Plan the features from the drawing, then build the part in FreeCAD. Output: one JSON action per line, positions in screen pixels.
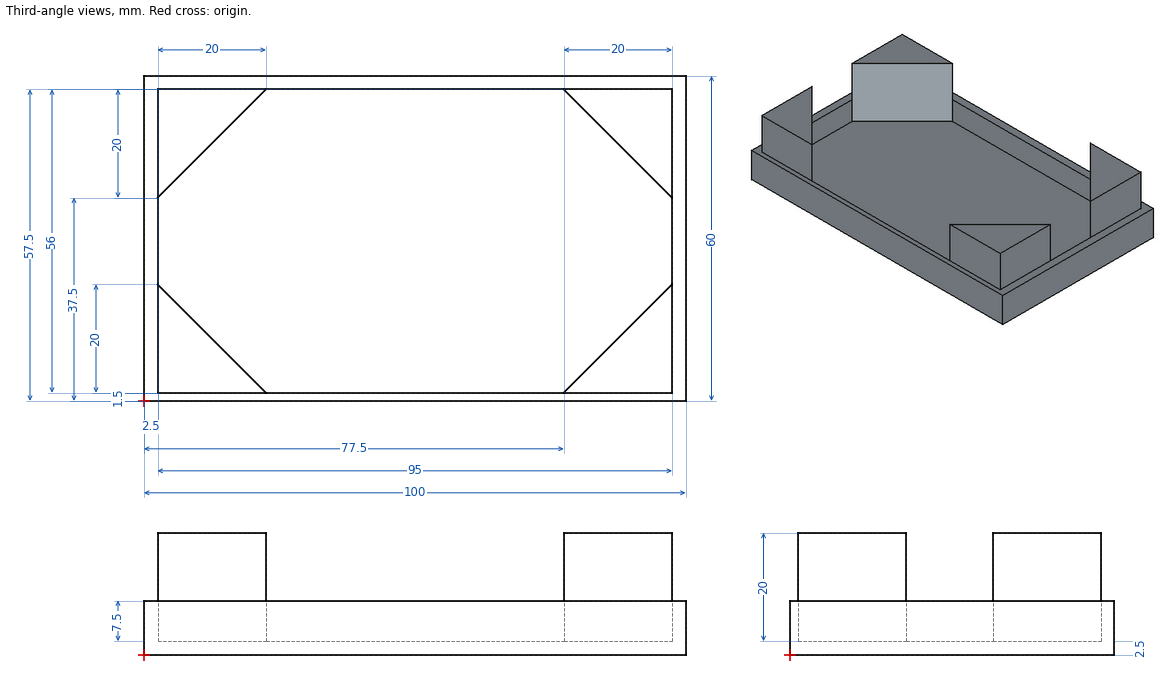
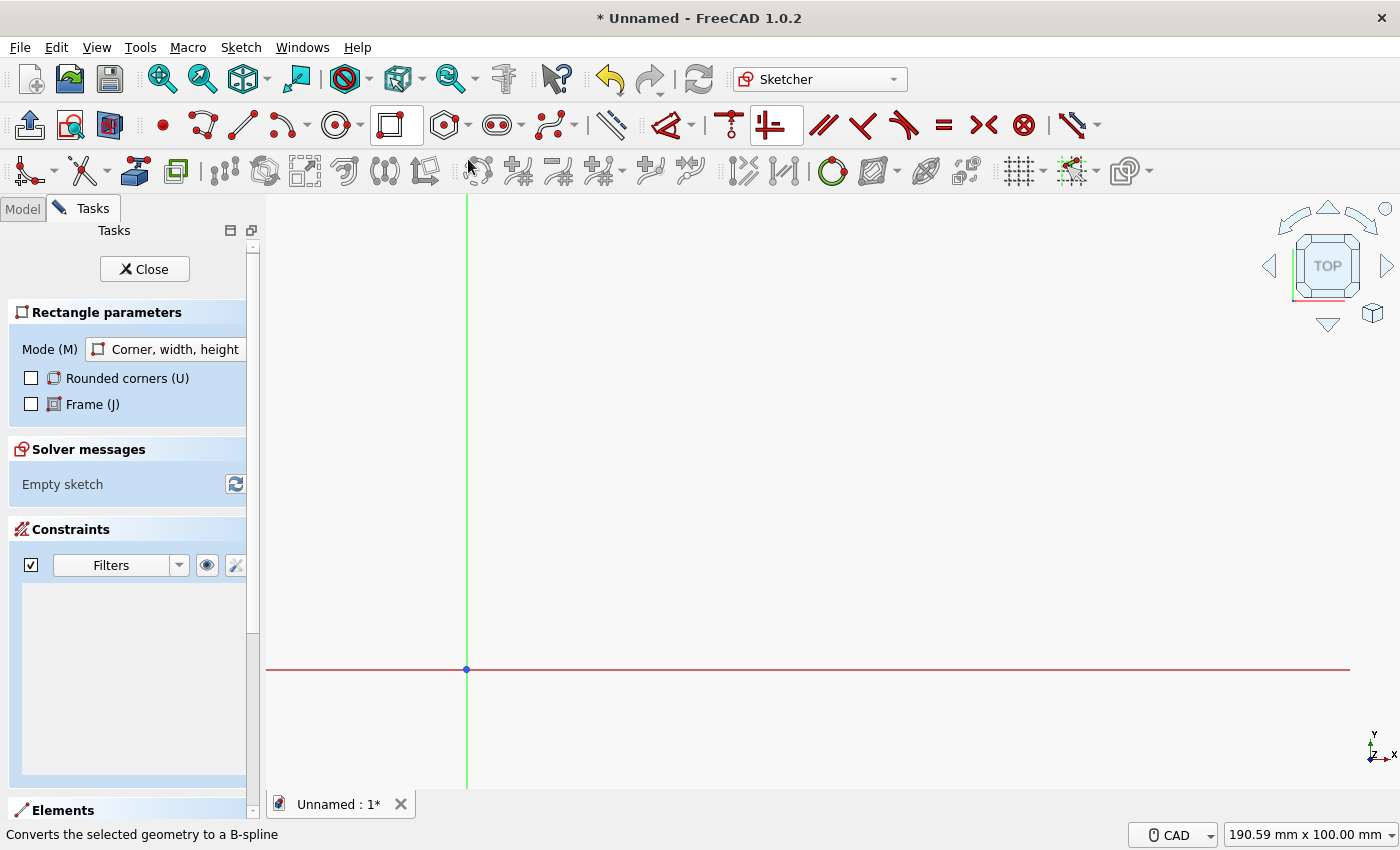
{"action": "left_click", "coordinate": [467, 670]}
{"action": "mouse_move", "coordinate": [1062, 313]}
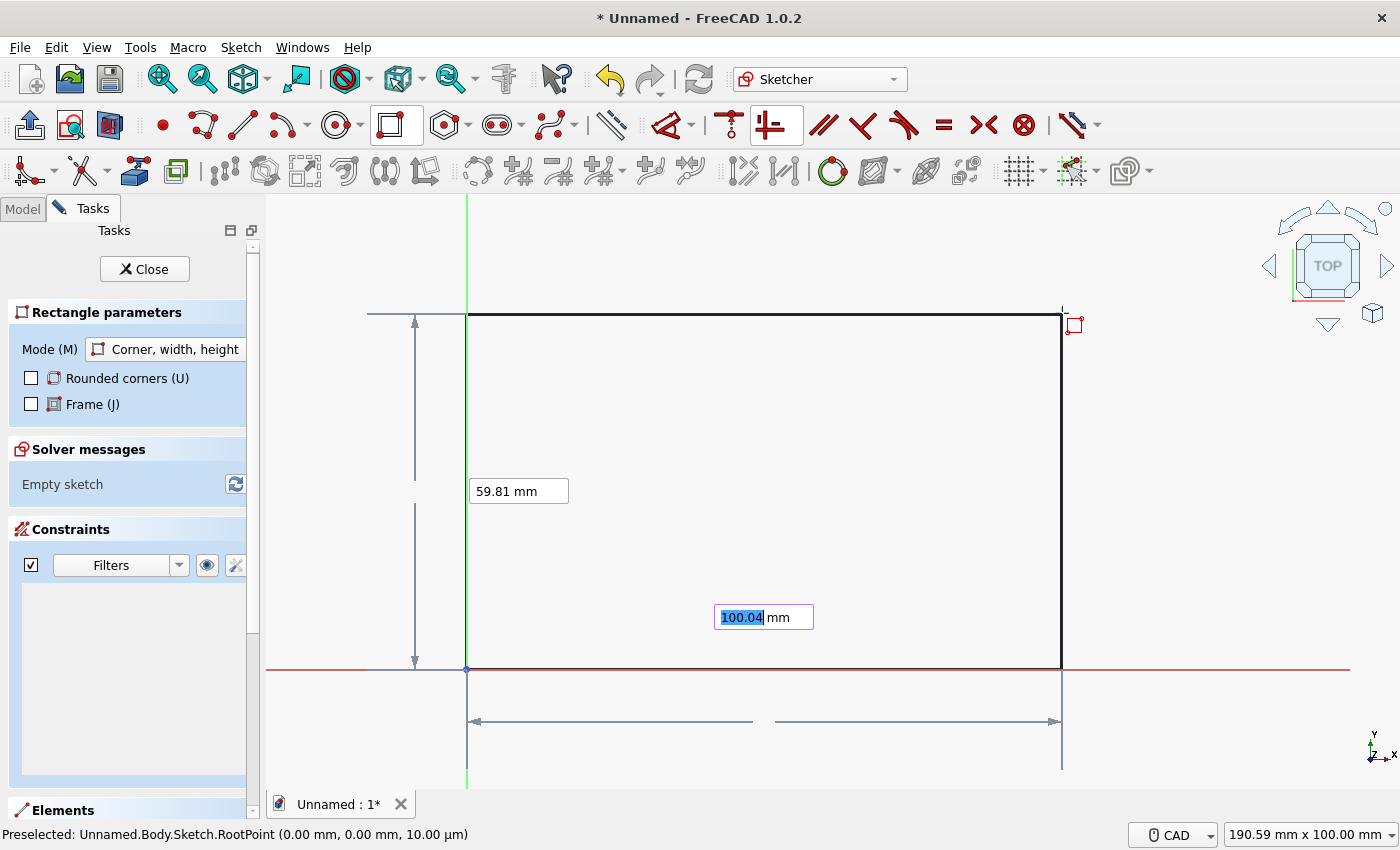
{"action": "type", "text": "100"}
{"action": "key", "text": "Tab"}
{"action": "type", "text": "60"}
{"action": "key", "text": "Return"}
{"action": "key", "text": "Escape"}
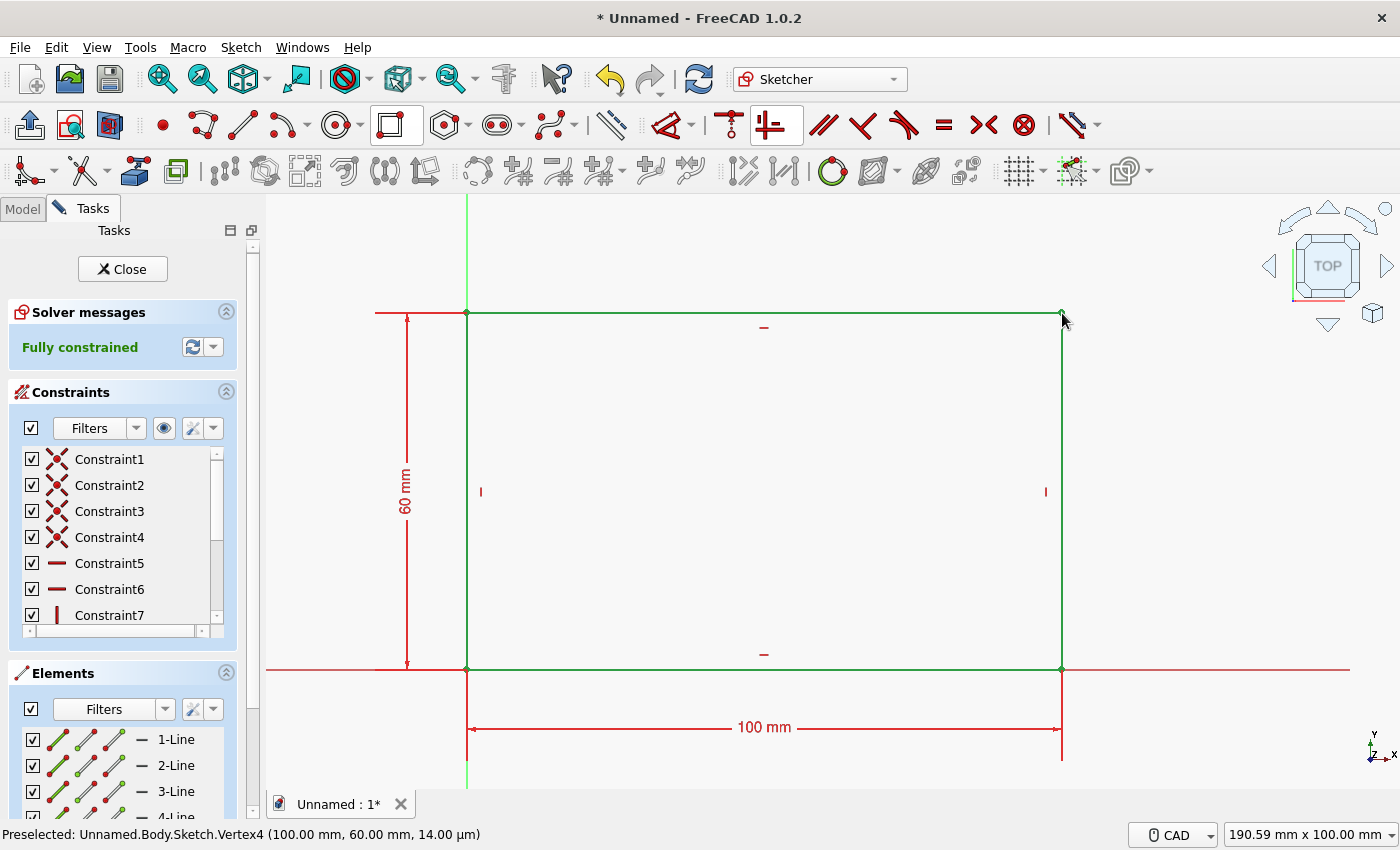
{"action": "left_click", "coordinate": [123, 269]}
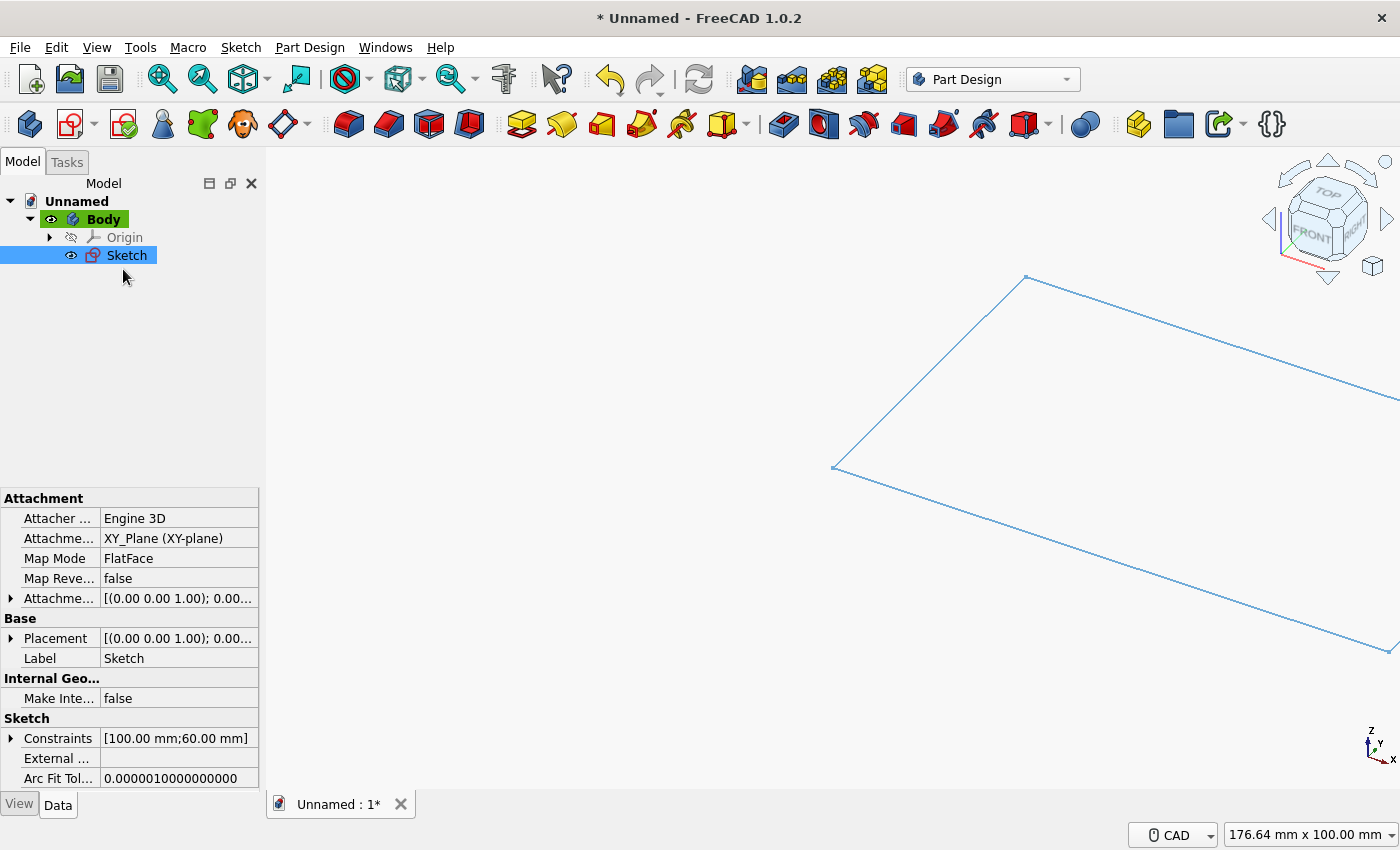
{"action": "left_click", "coordinate": [522, 124]}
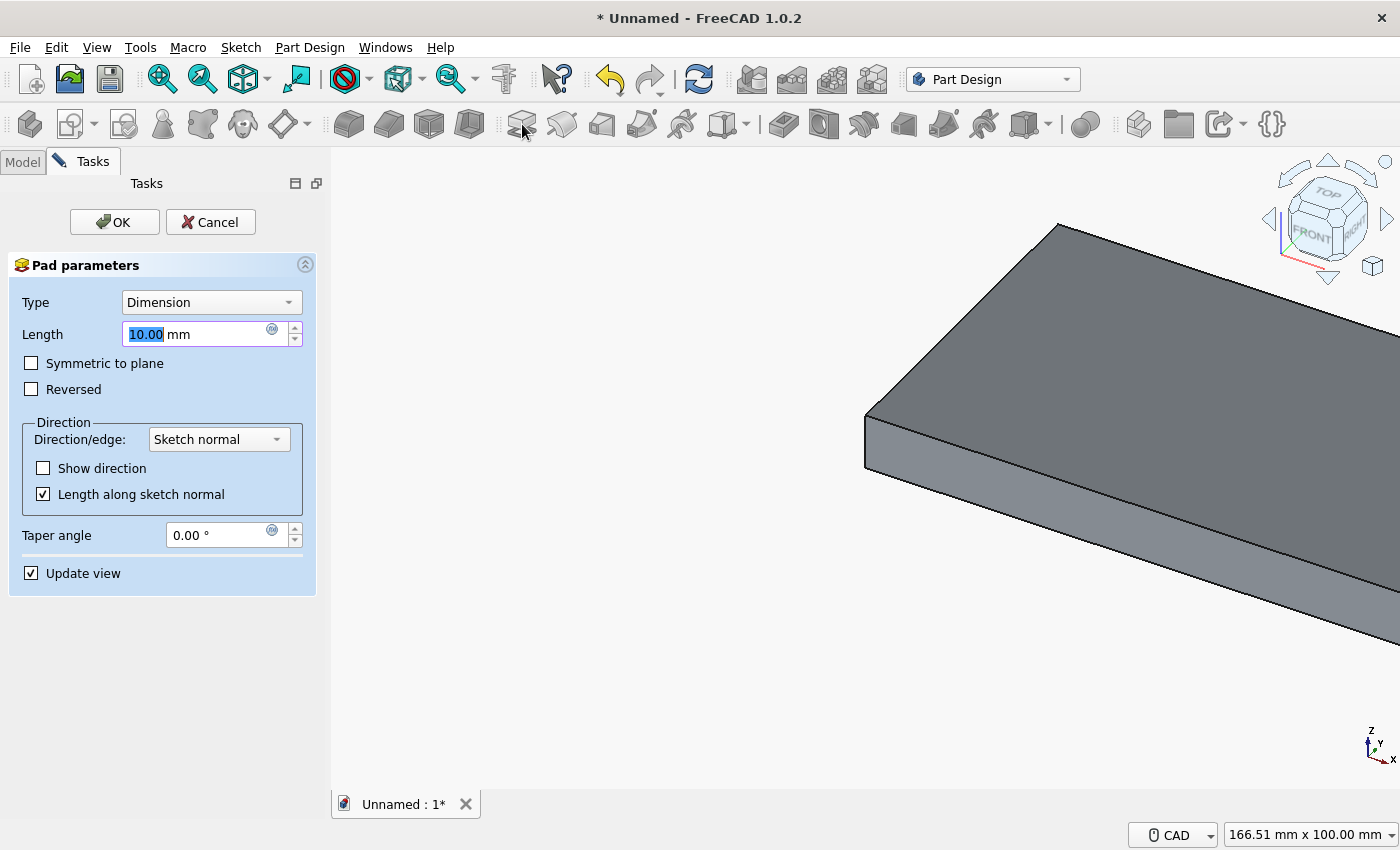
{"action": "type", "text": "2.5"}
{"action": "key", "text": "Tab"}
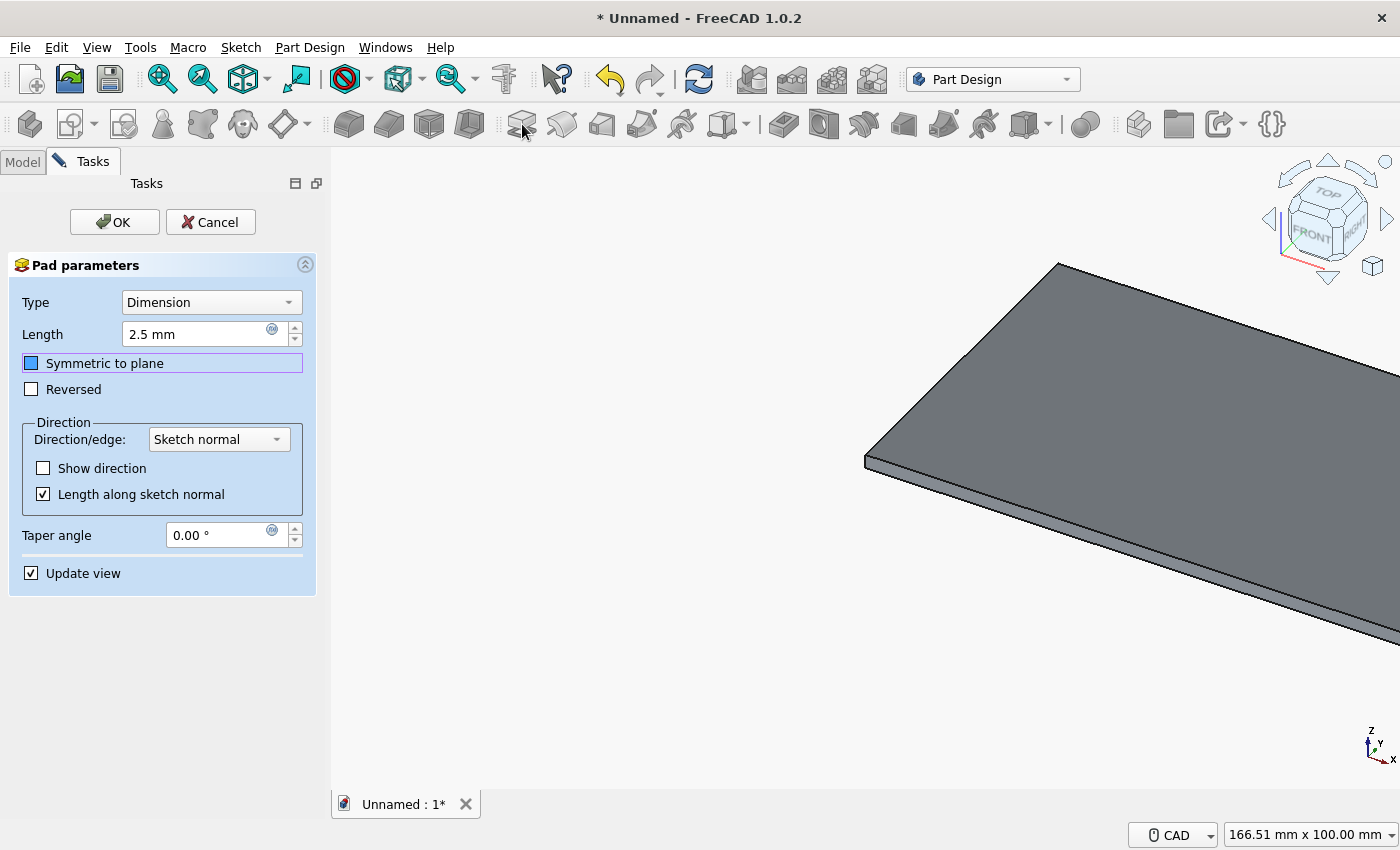
{"action": "left_click", "coordinate": [115, 222]}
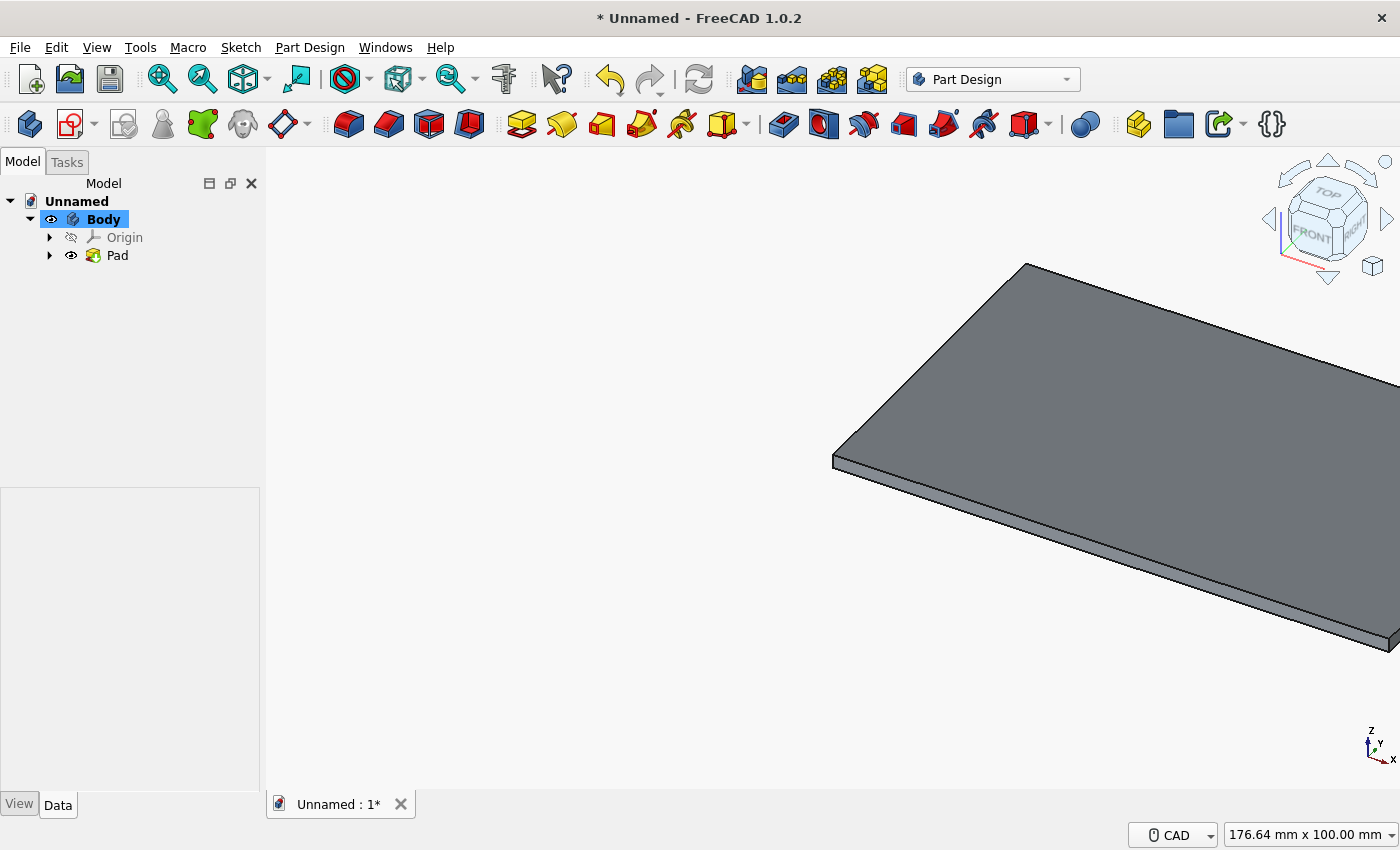
{"action": "left_click", "coordinate": [164, 80]}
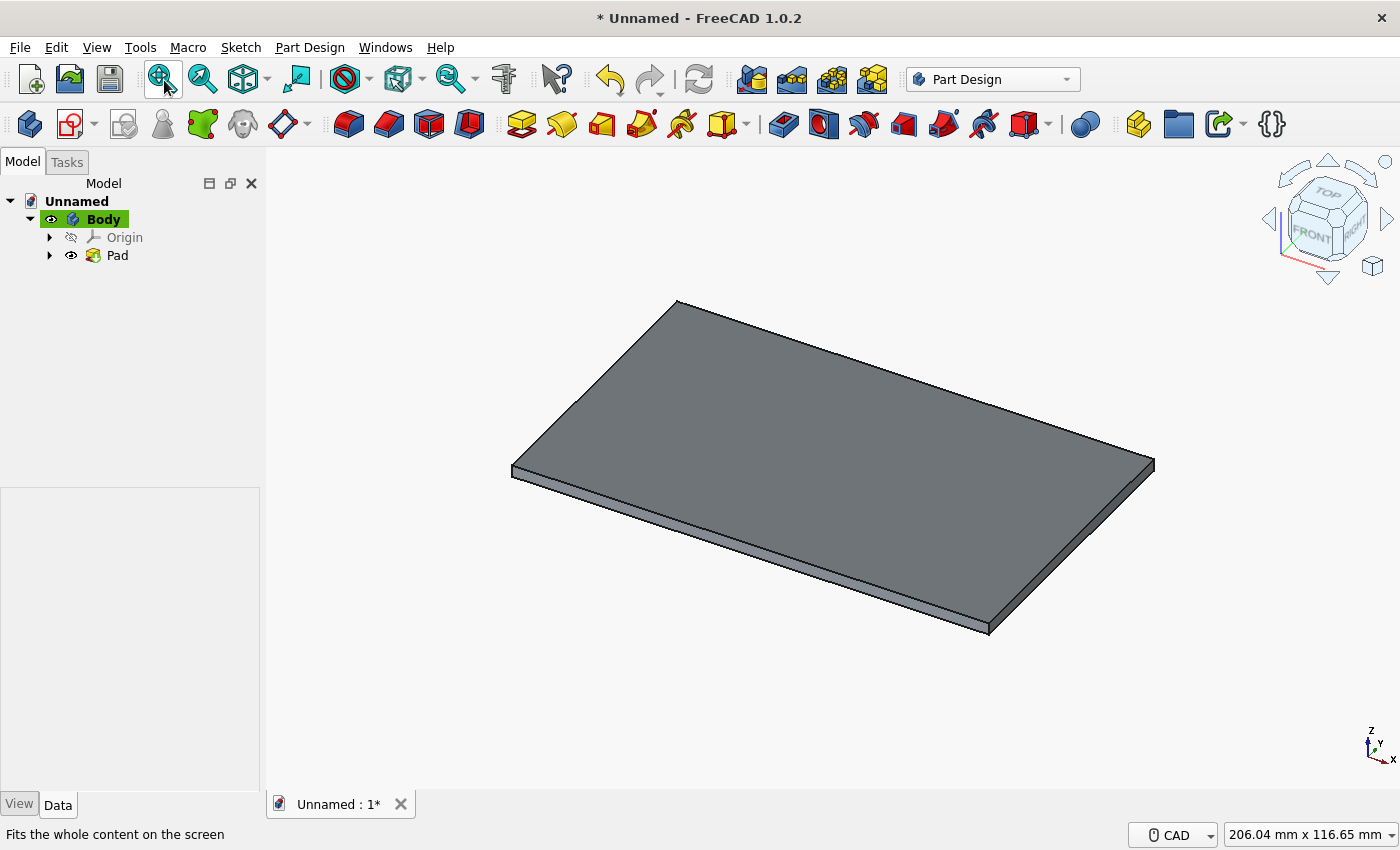
{"action": "left_click", "coordinate": [901, 484]}